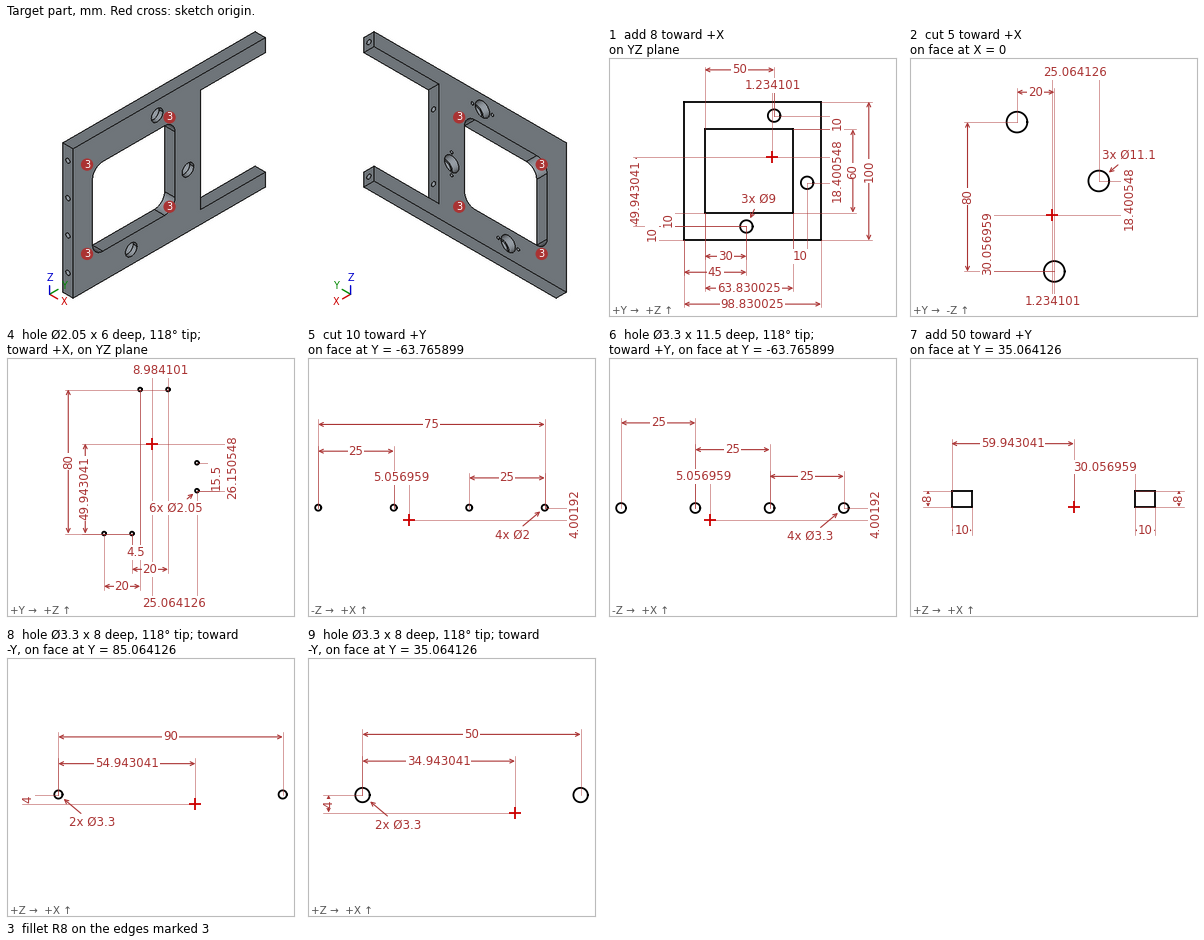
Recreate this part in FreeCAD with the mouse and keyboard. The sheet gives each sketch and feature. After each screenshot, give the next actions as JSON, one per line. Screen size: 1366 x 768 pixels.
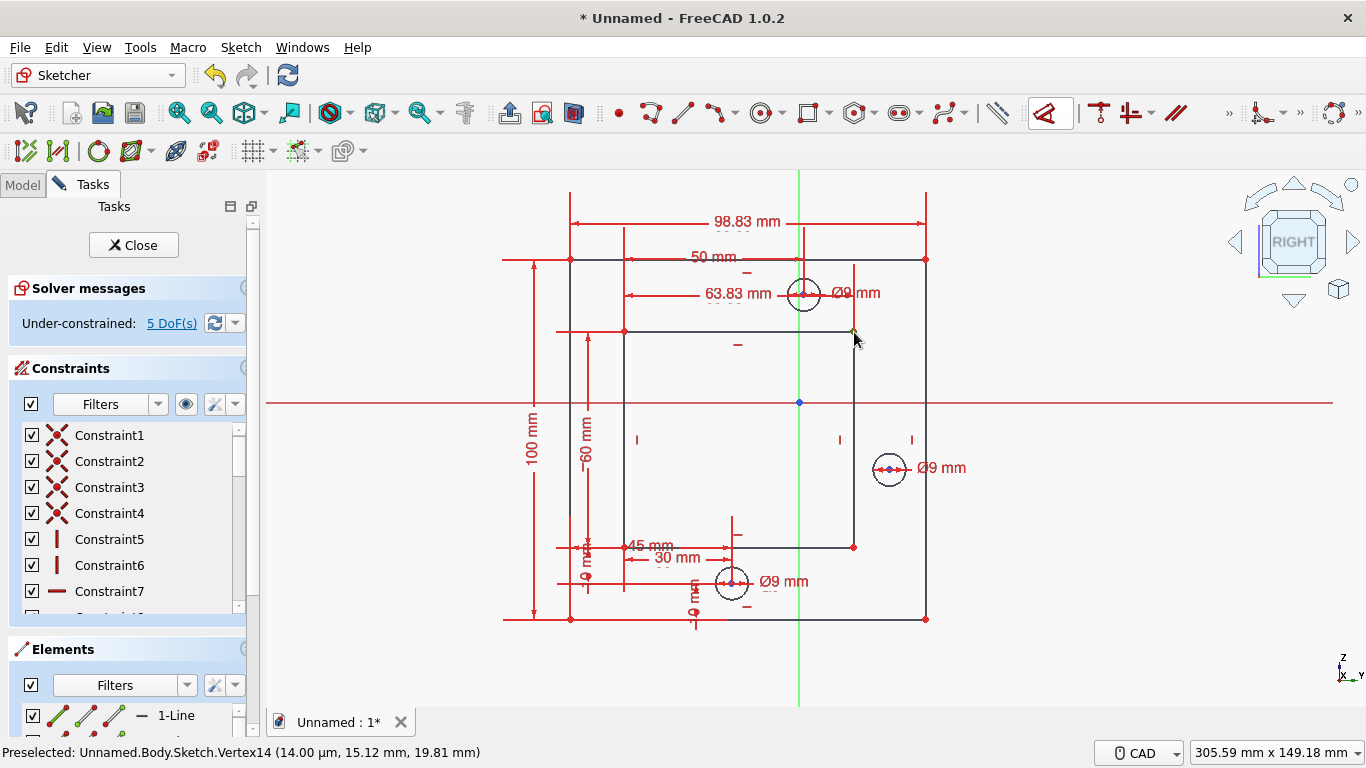
{"action": "left_click", "coordinate": [804, 295]}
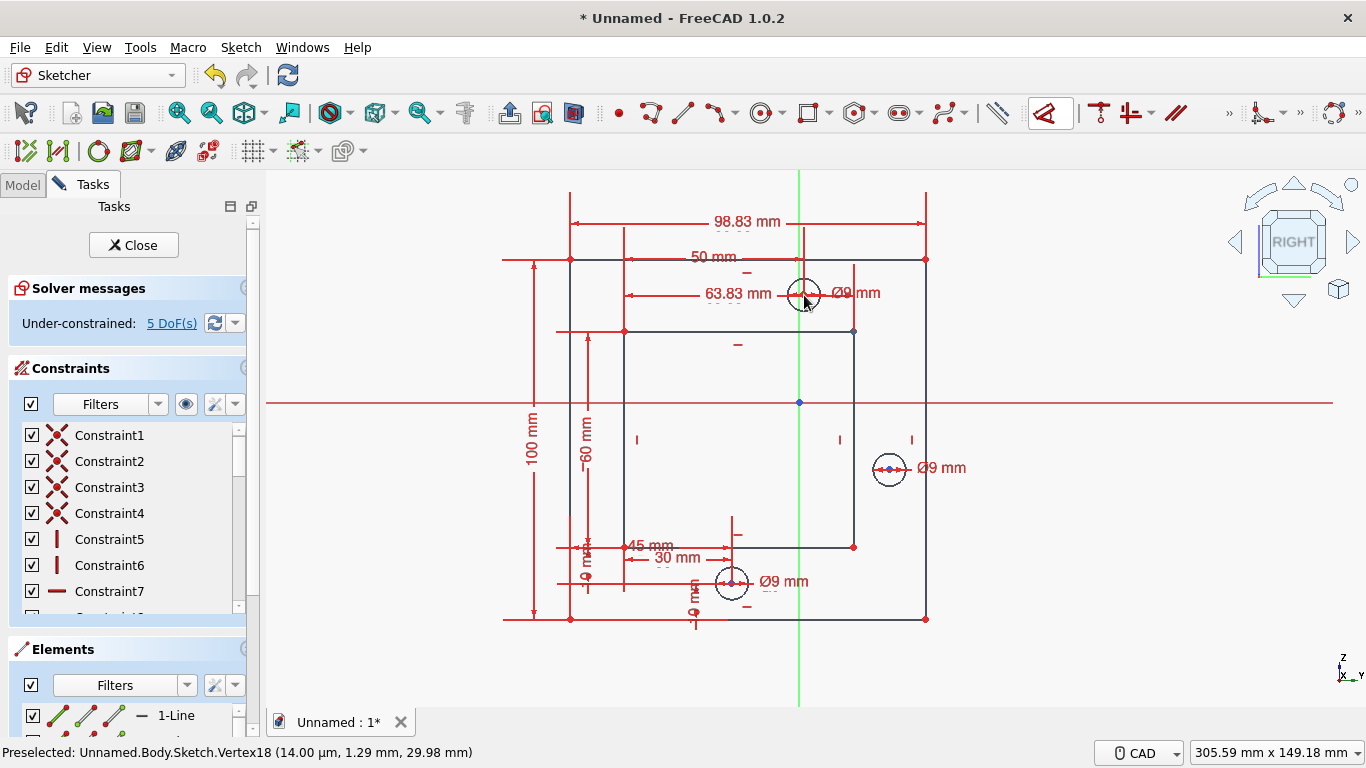
{"action": "key", "text": "i"}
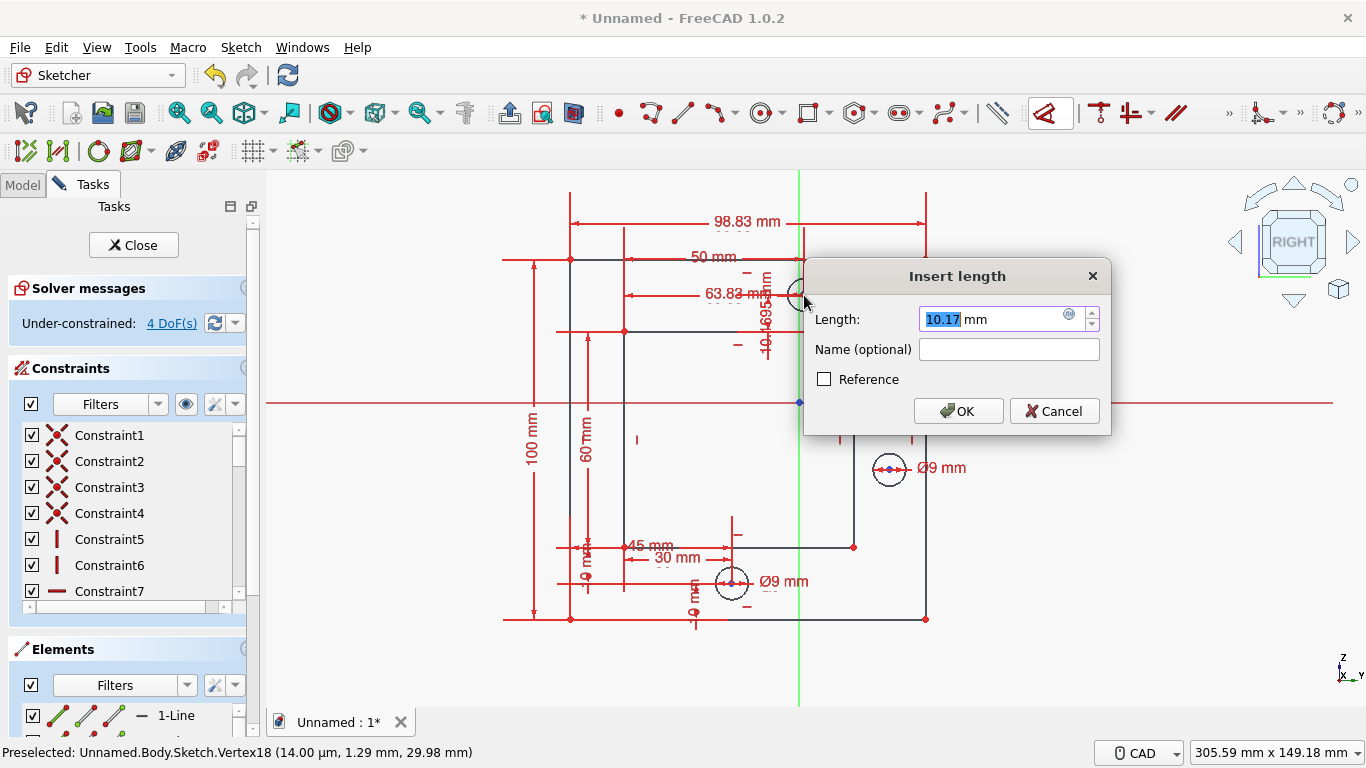
{"action": "type", "text": "10"}
{"action": "key", "text": "Return"}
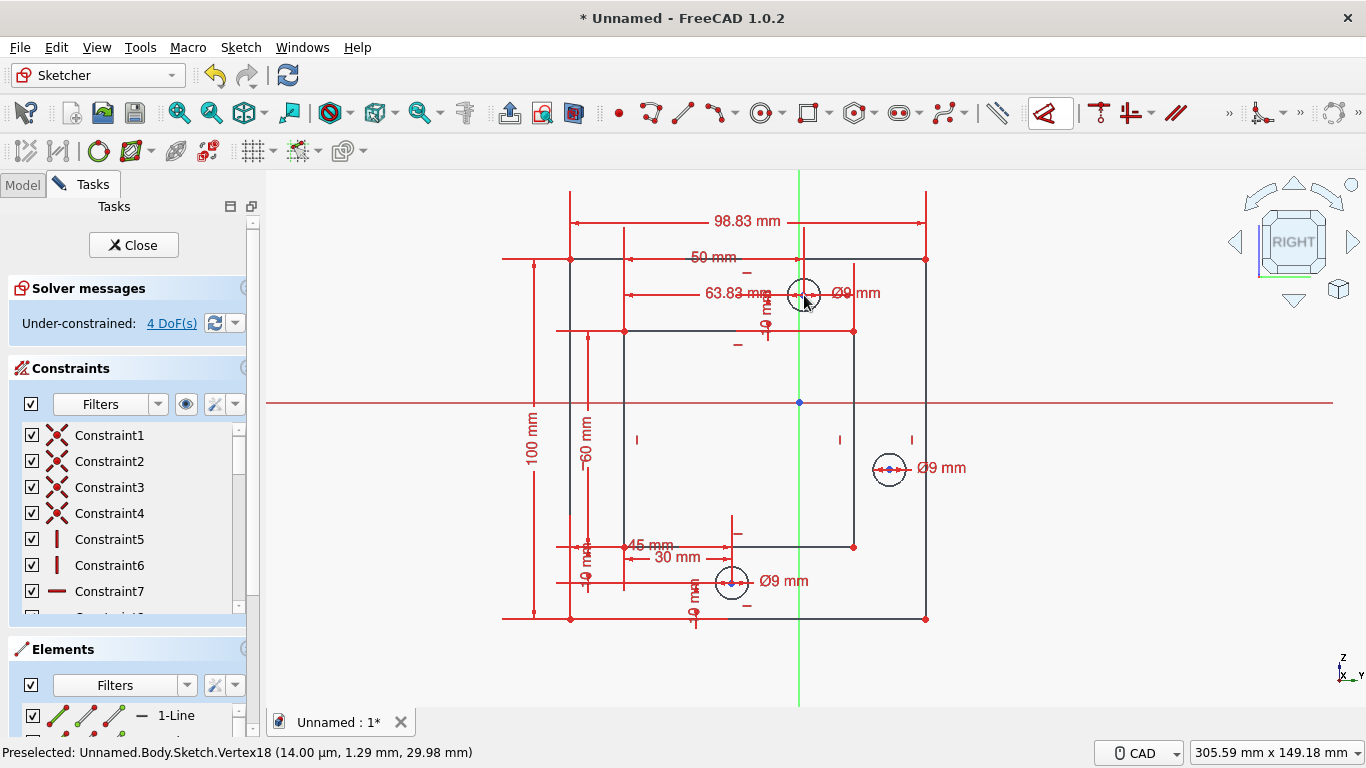
{"action": "left_click", "coordinate": [854, 547]}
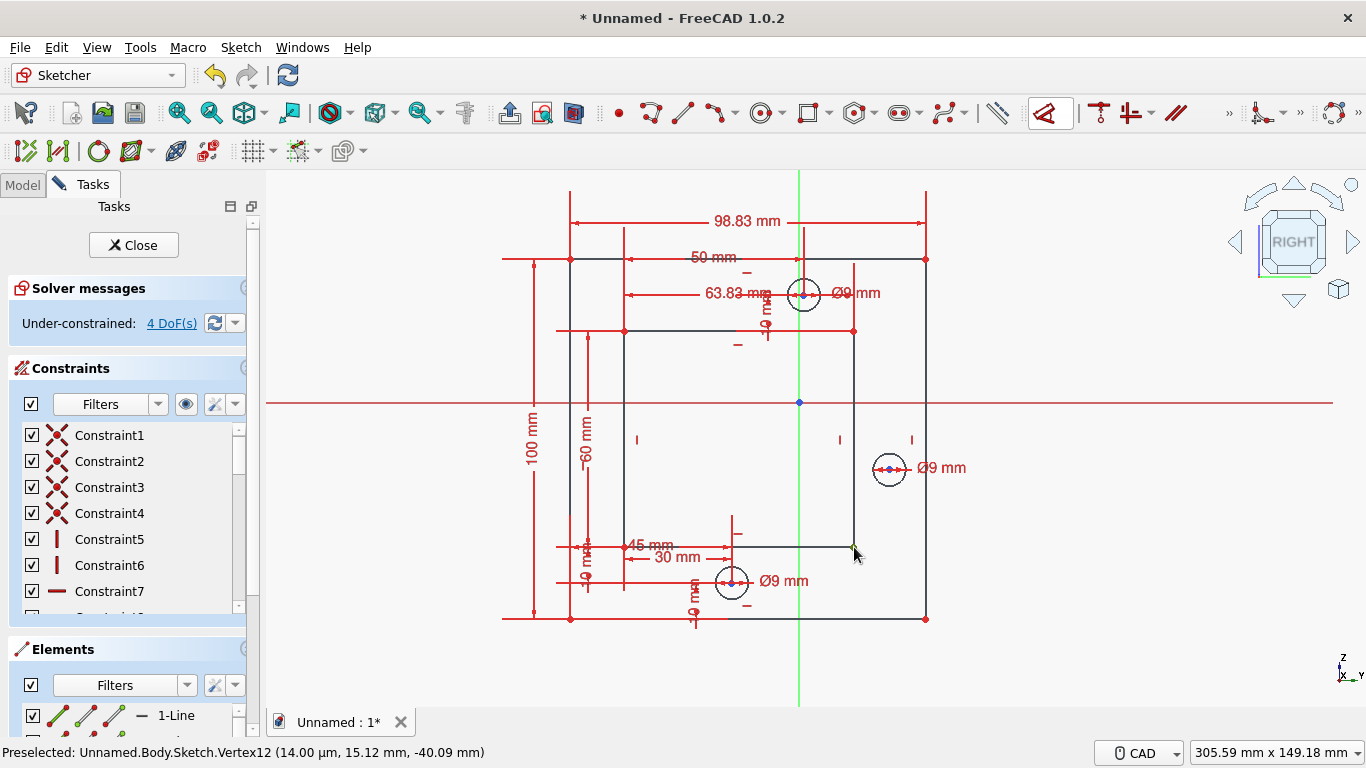
{"action": "left_click", "coordinate": [890, 470]}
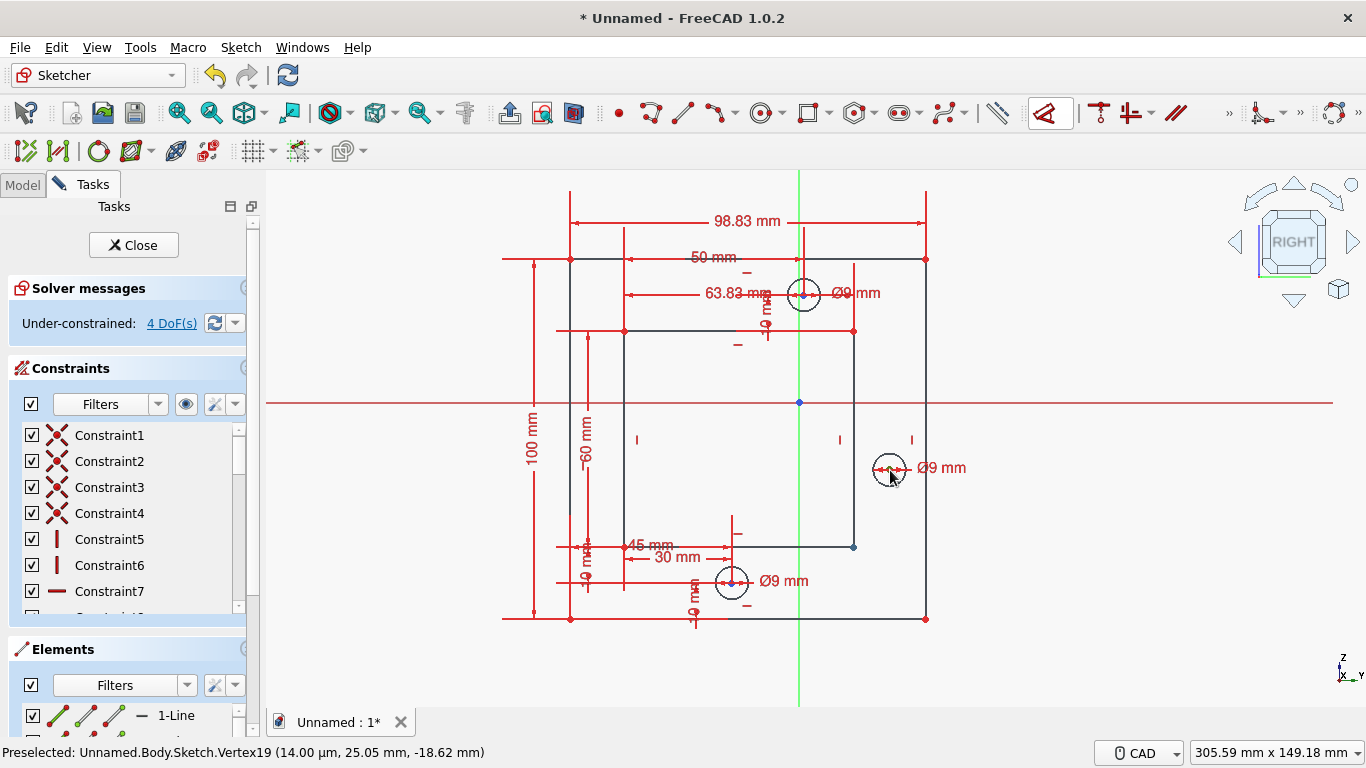
{"action": "left_click", "coordinate": [1068, 114]}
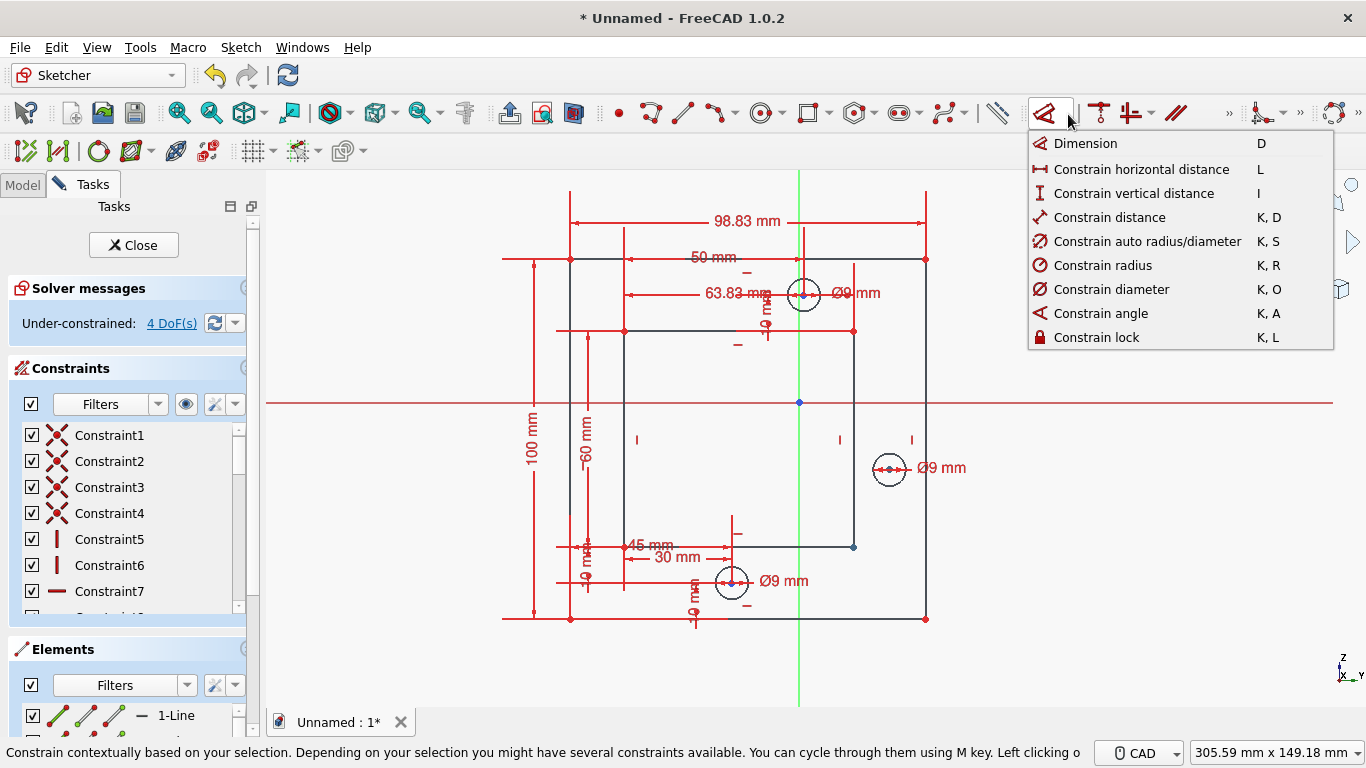
{"action": "left_click", "coordinate": [1181, 169]}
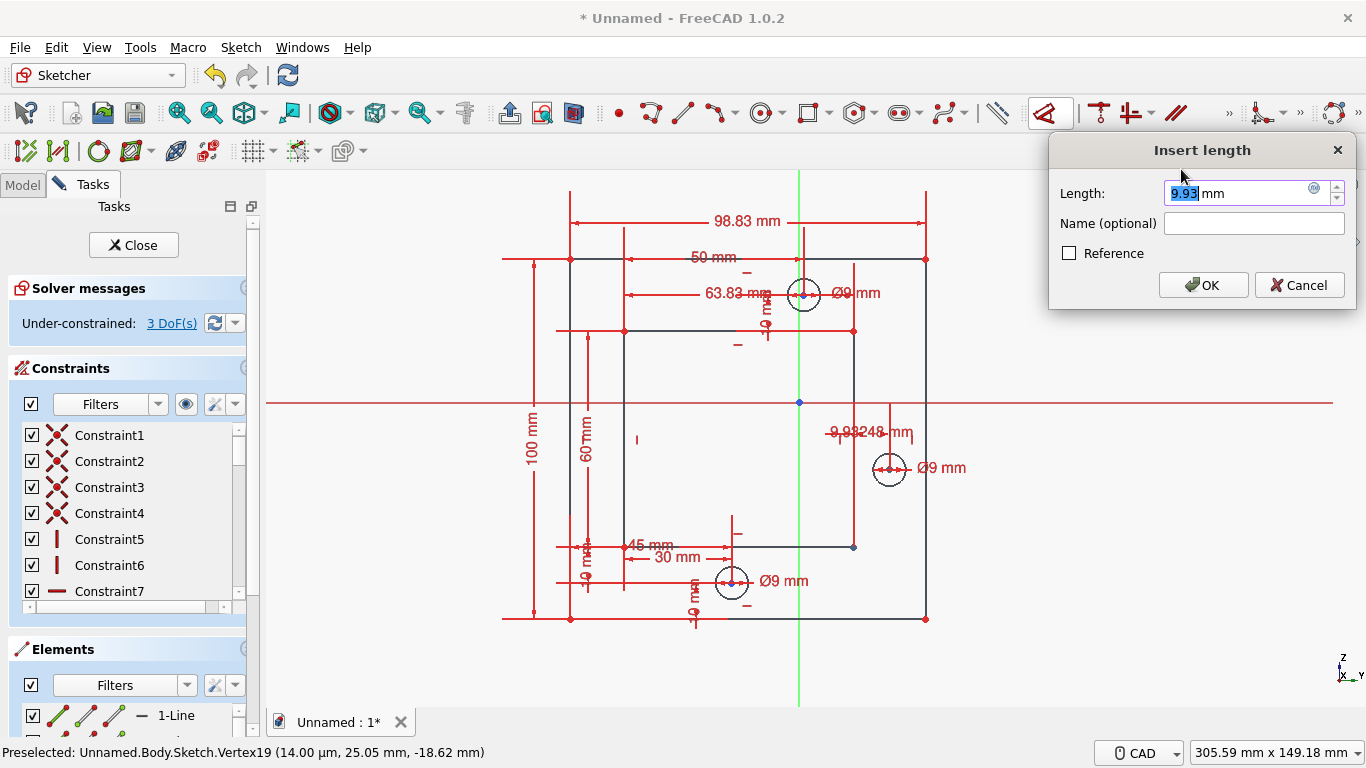
{"action": "type", "text": "10"}
{"action": "key", "text": "Return"}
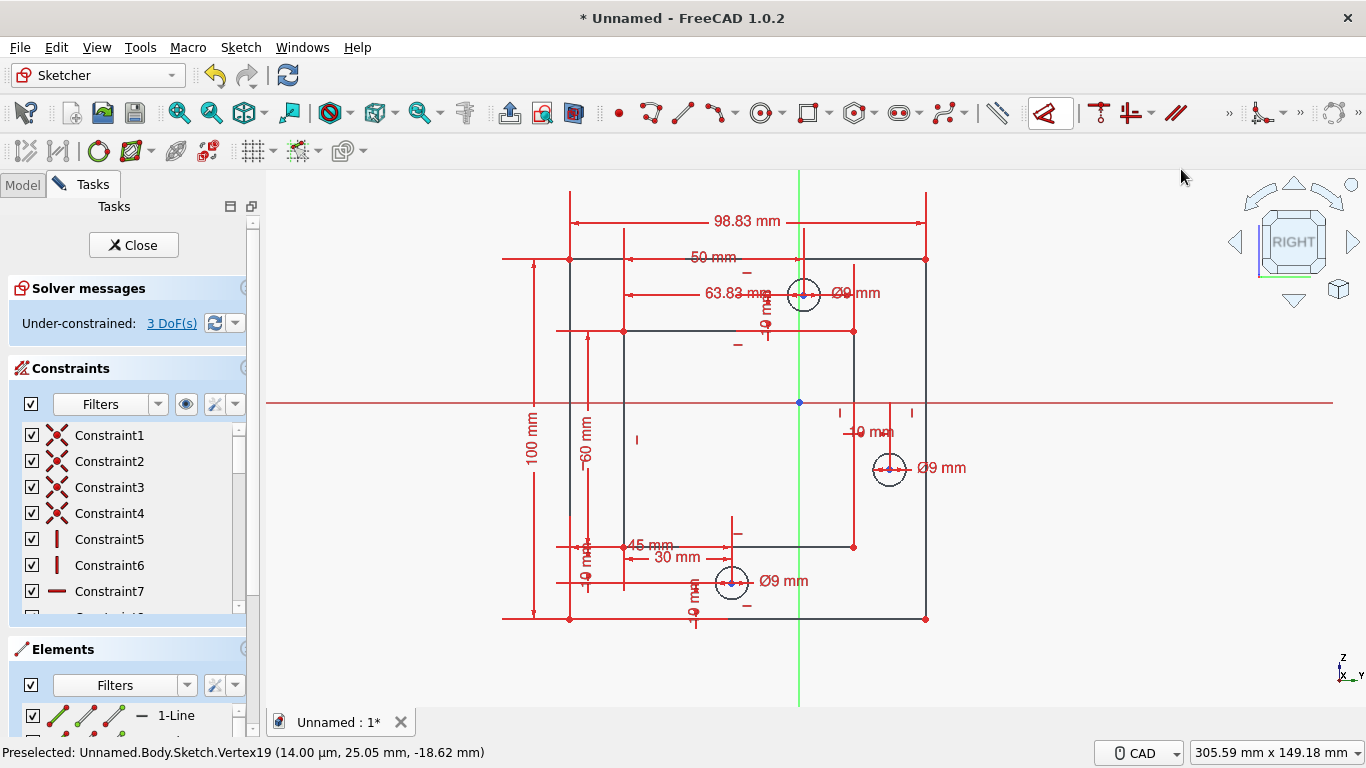
{"action": "scroll", "coordinate": [804, 295], "scroll_direction": "up", "scroll_amount": 11}